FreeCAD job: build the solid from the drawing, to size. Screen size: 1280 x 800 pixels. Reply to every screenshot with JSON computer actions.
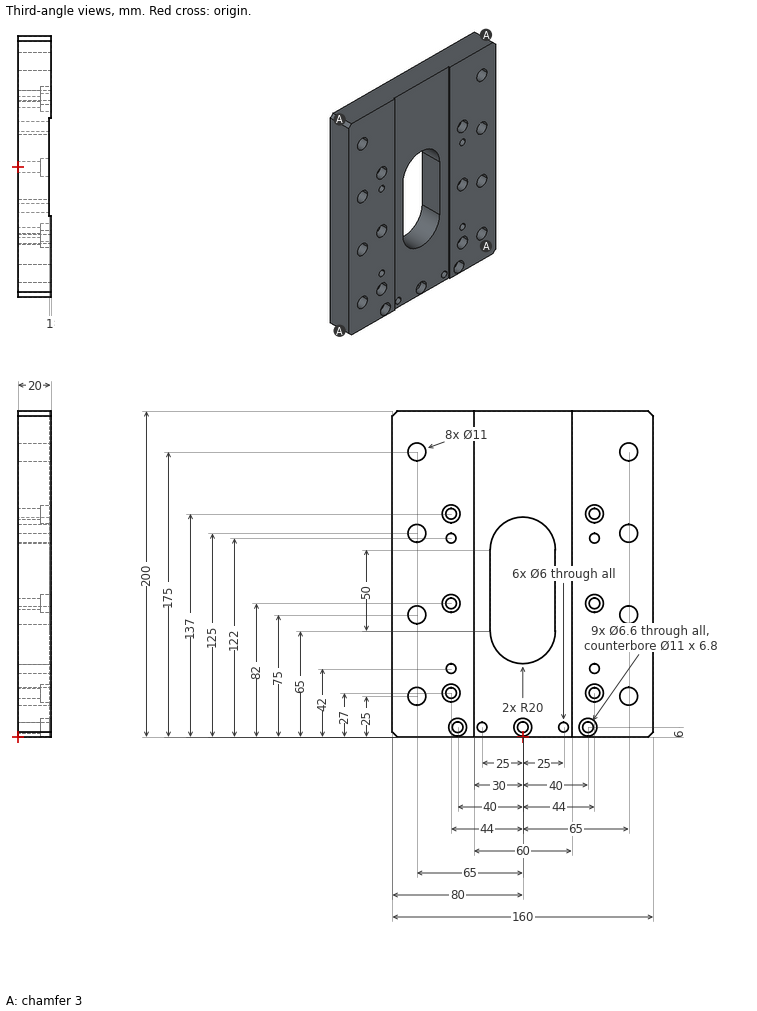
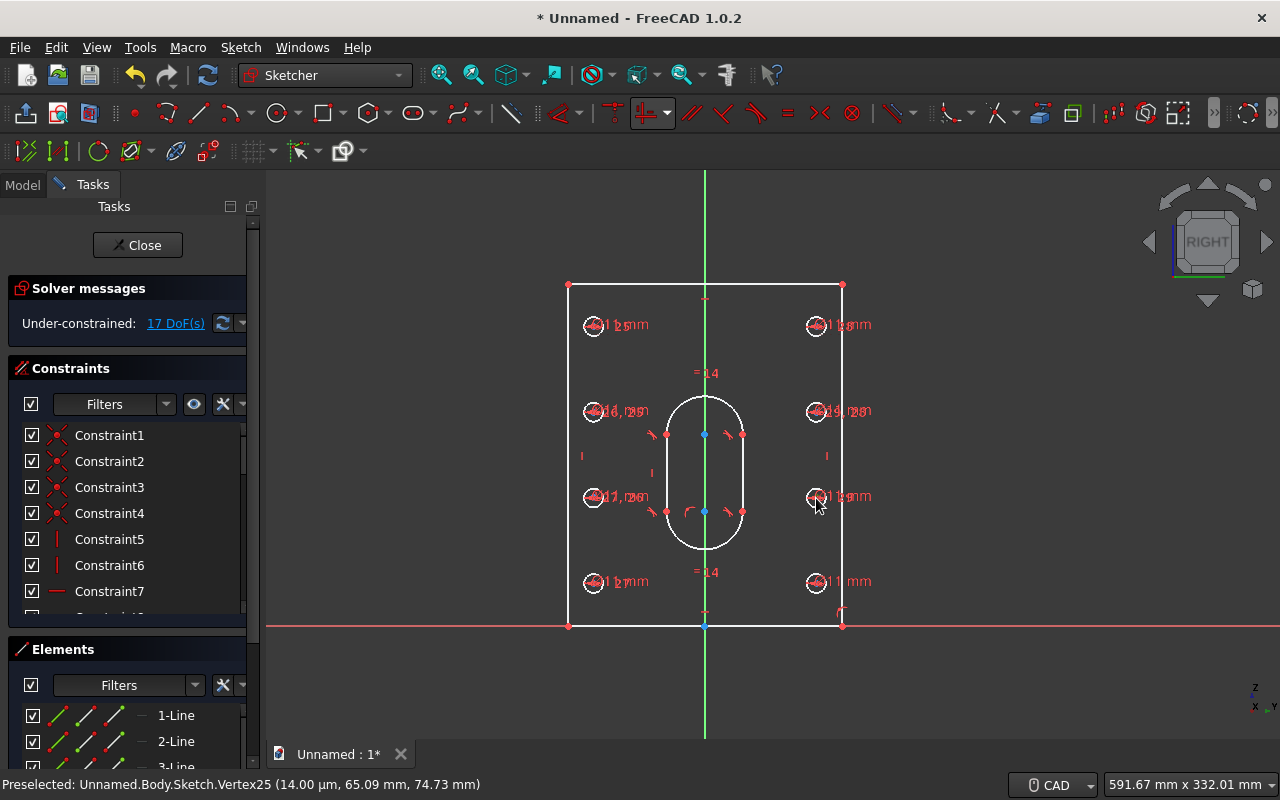
{"action": "left_click", "coordinate": [816, 583]}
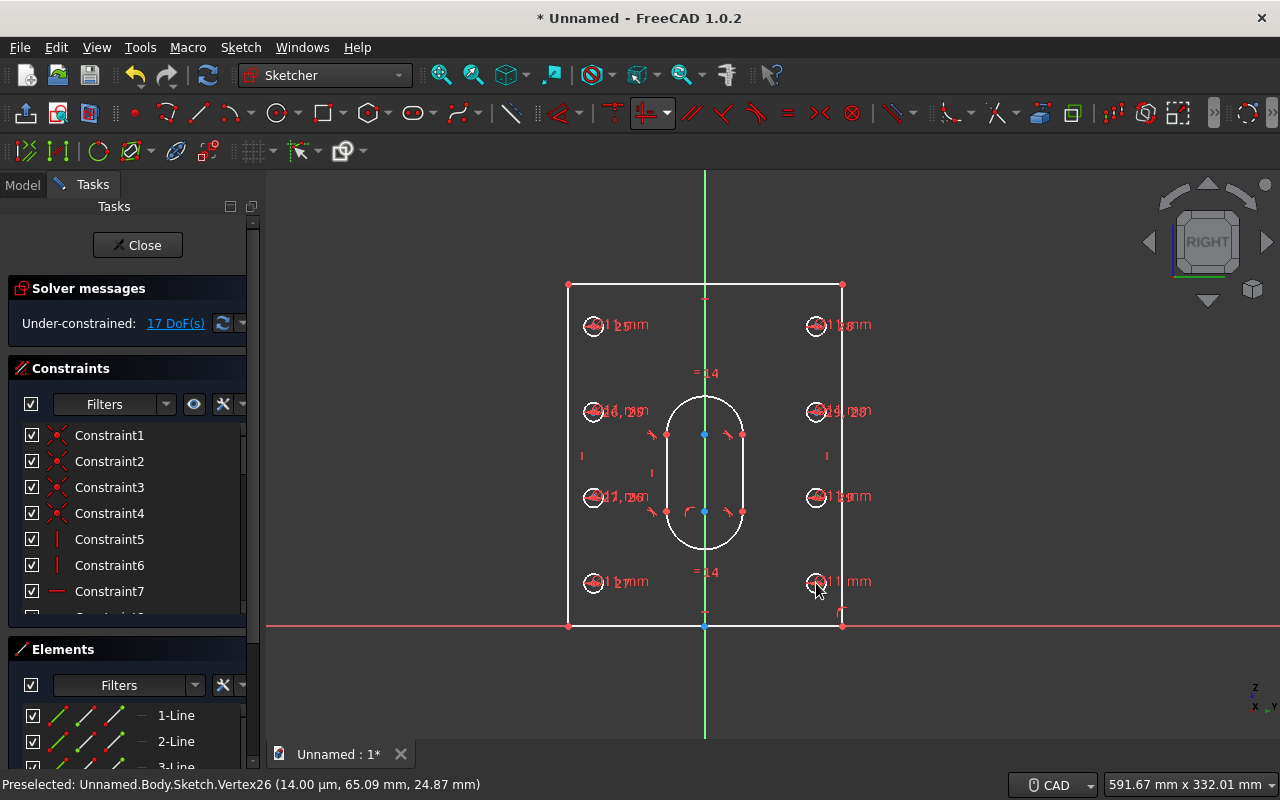
{"action": "key", "text": "v"}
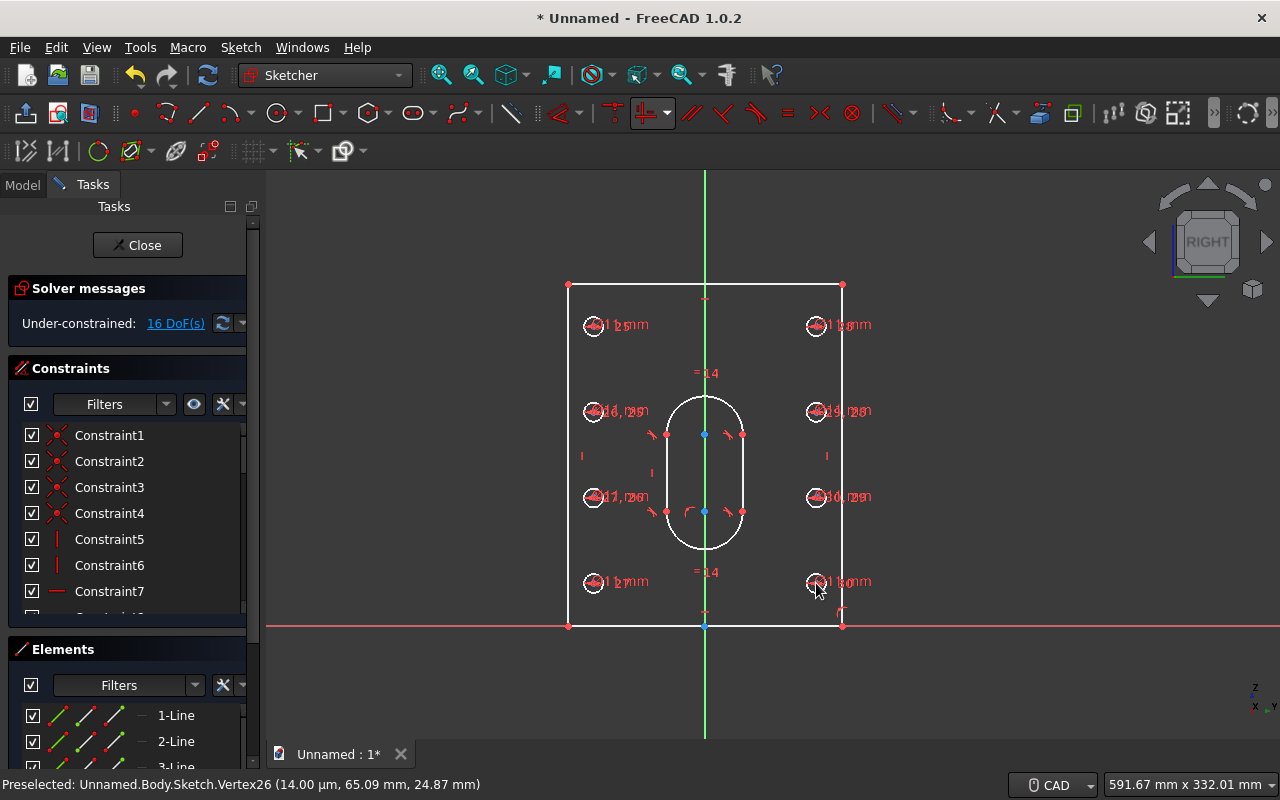
{"action": "key", "text": "d"}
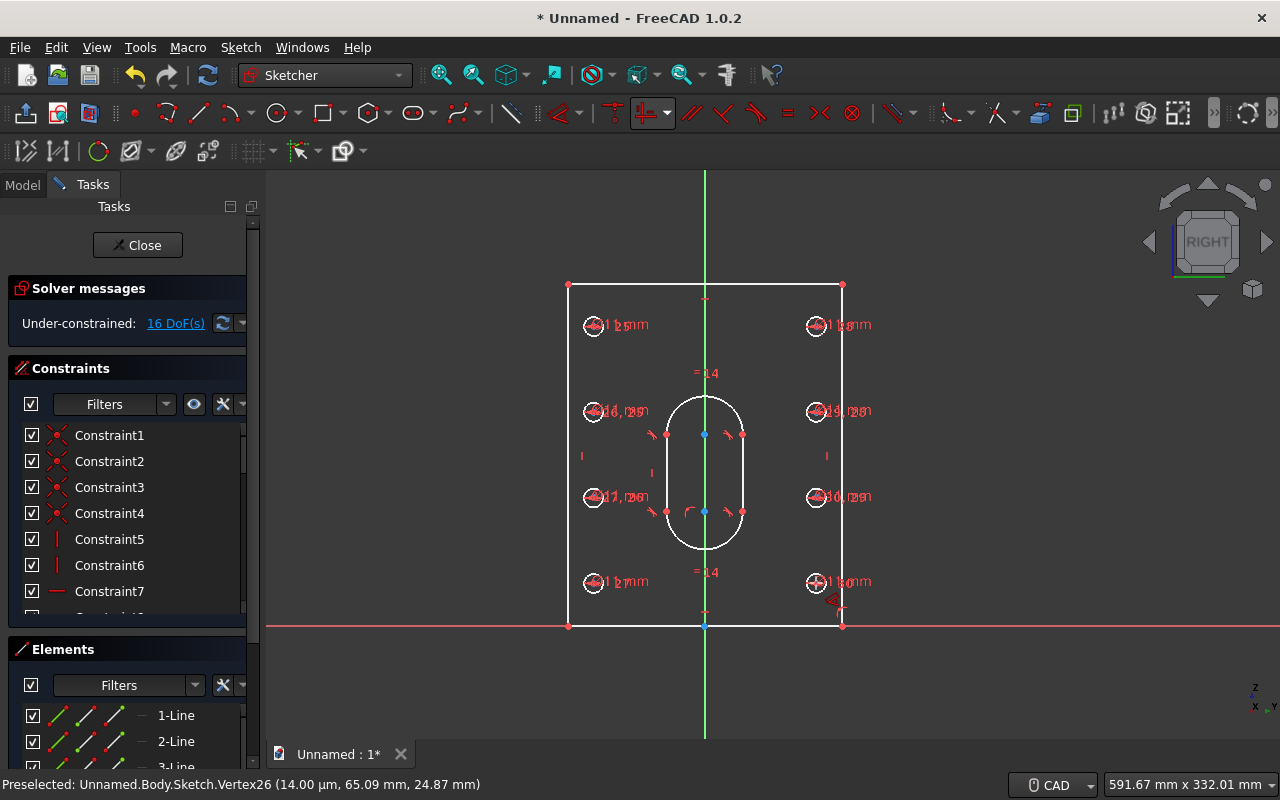
{"action": "left_click", "coordinate": [682, 542]}
{"action": "left_click", "coordinate": [663, 568]}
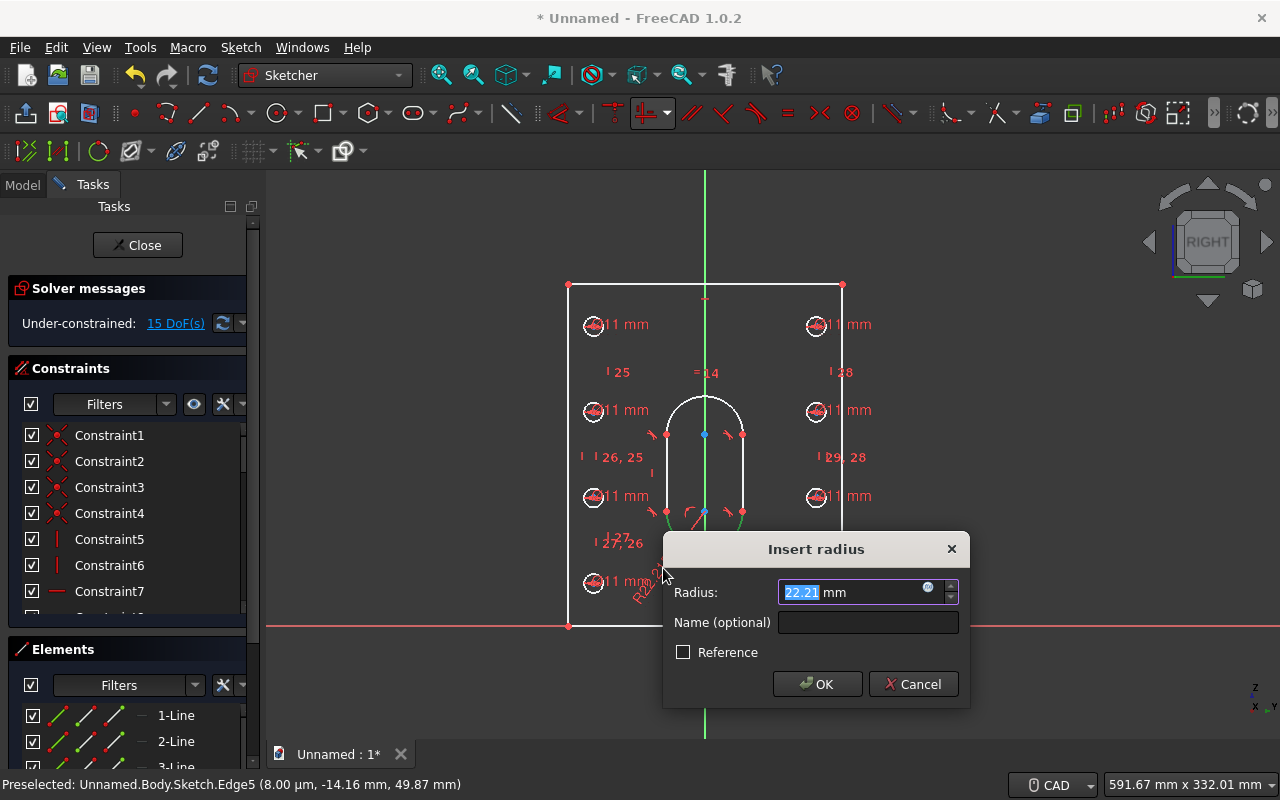
{"action": "type", "text": "20"}
{"action": "key", "text": "Return"}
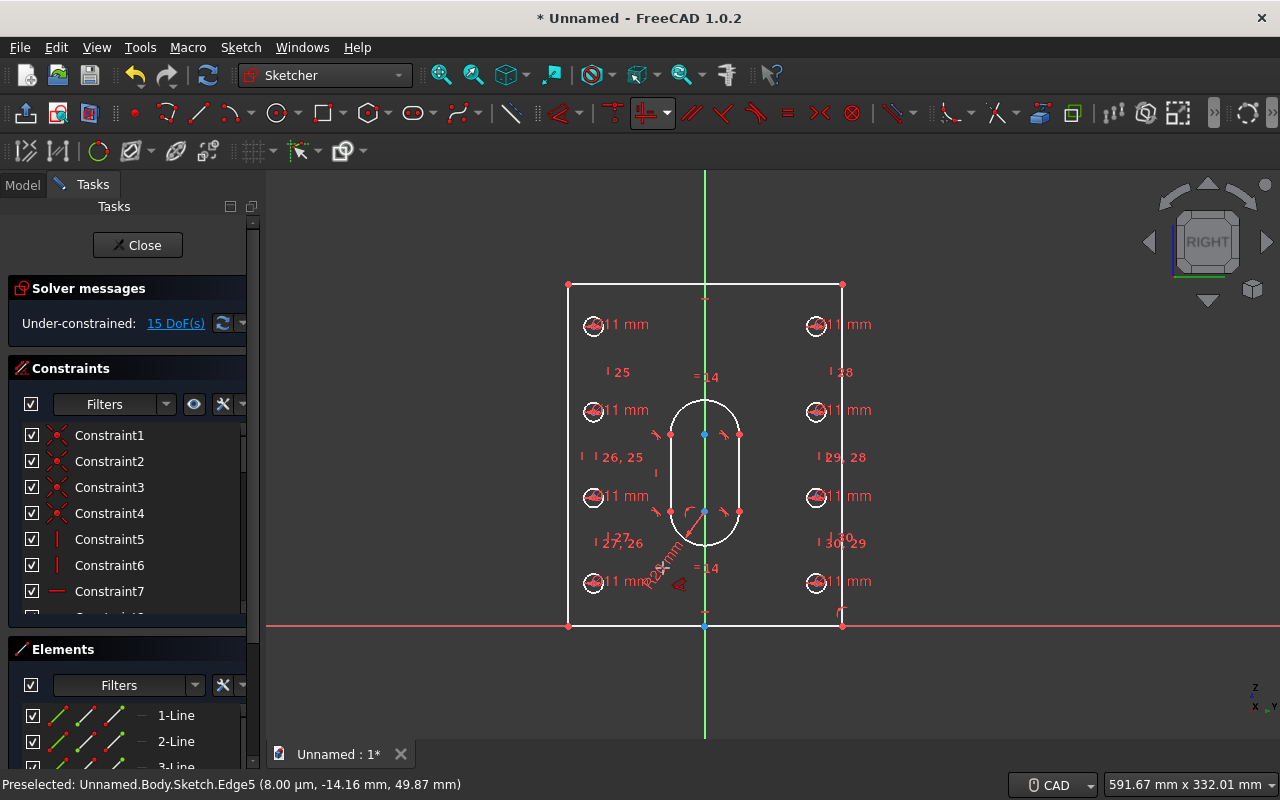
{"action": "left_click", "coordinate": [671, 488]}
{"action": "left_click", "coordinate": [637, 473]}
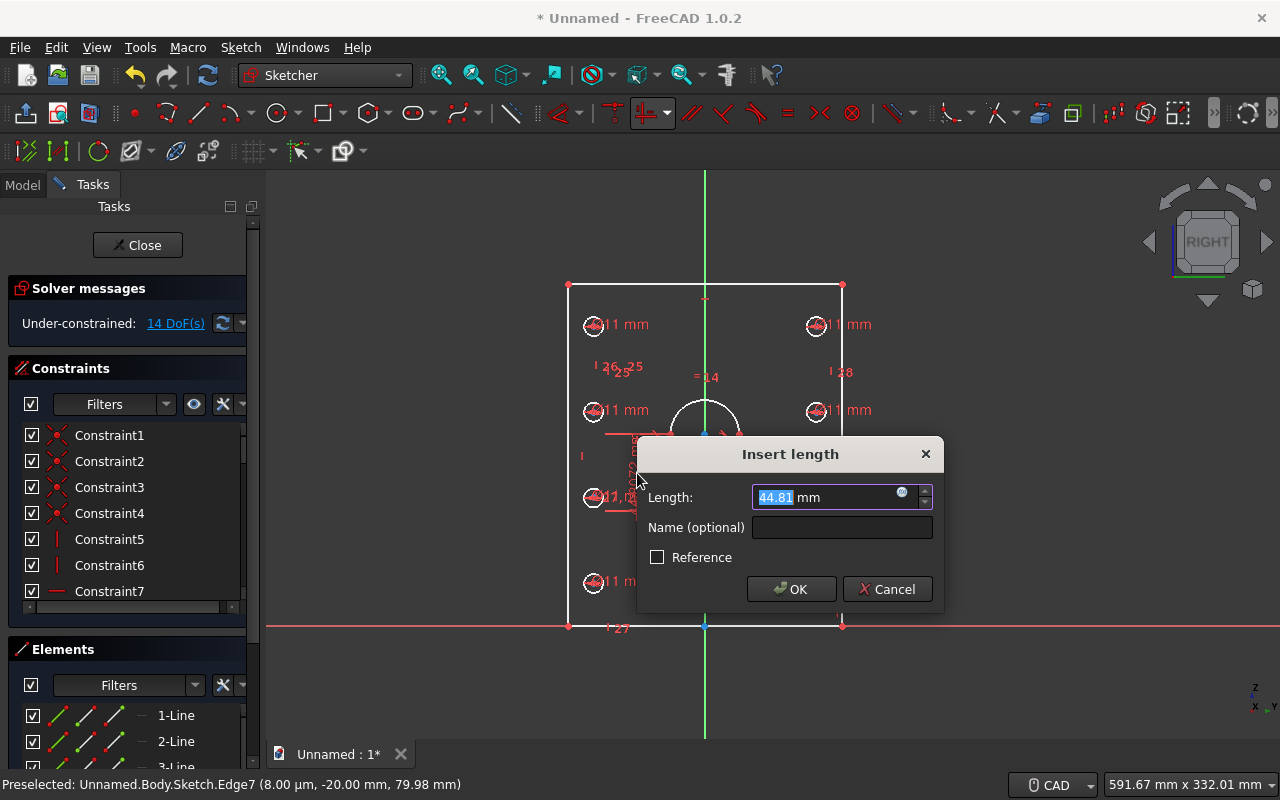
{"action": "type", "text": "50"}
{"action": "key", "text": "Return"}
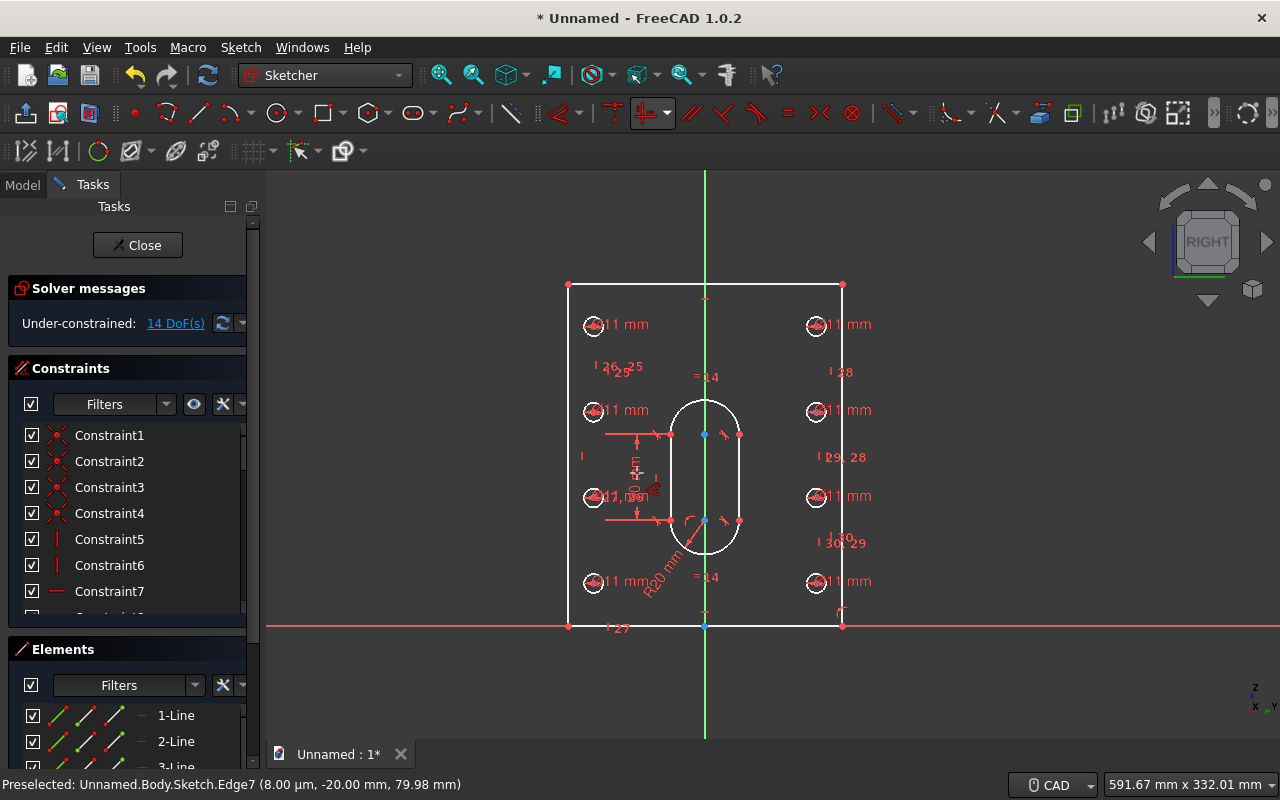
{"action": "left_click", "coordinate": [594, 327]}
{"action": "left_click", "coordinate": [649, 660]}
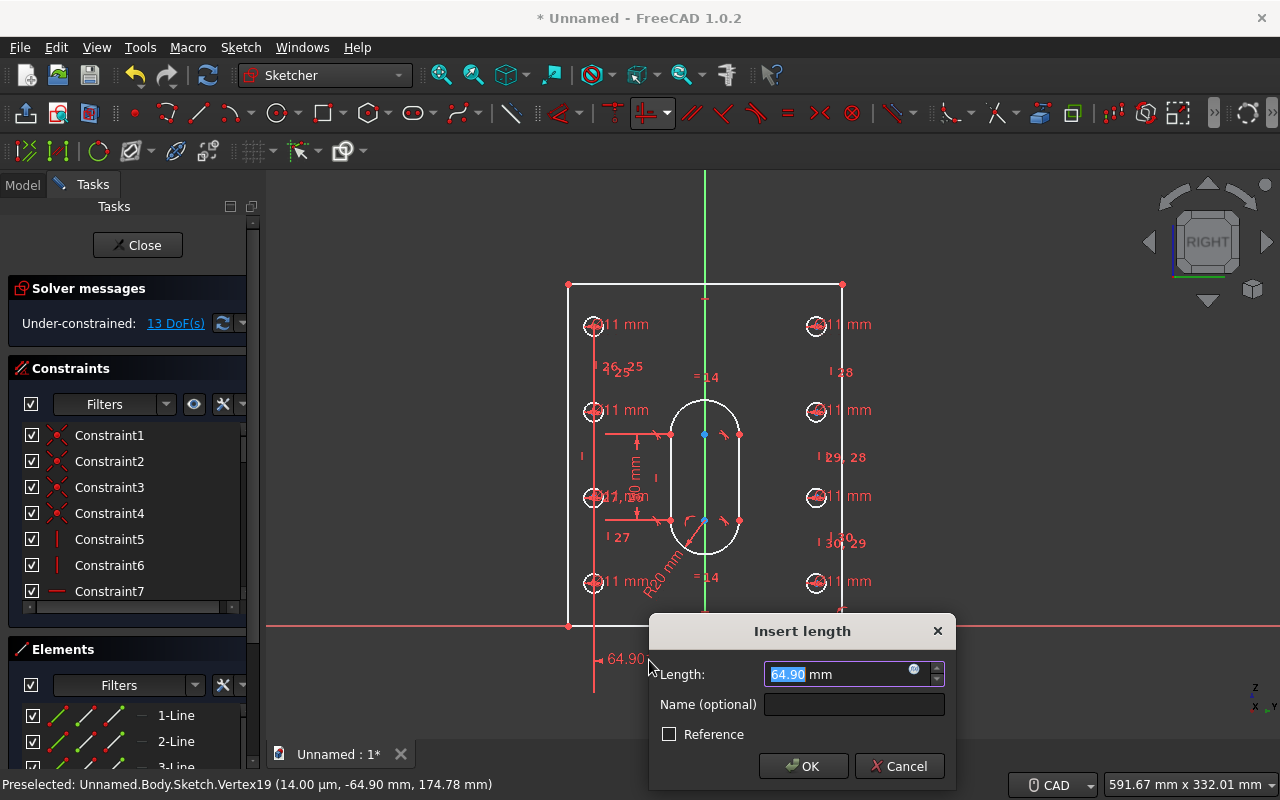
{"action": "type", "text": "65"}
{"action": "key", "text": "Return"}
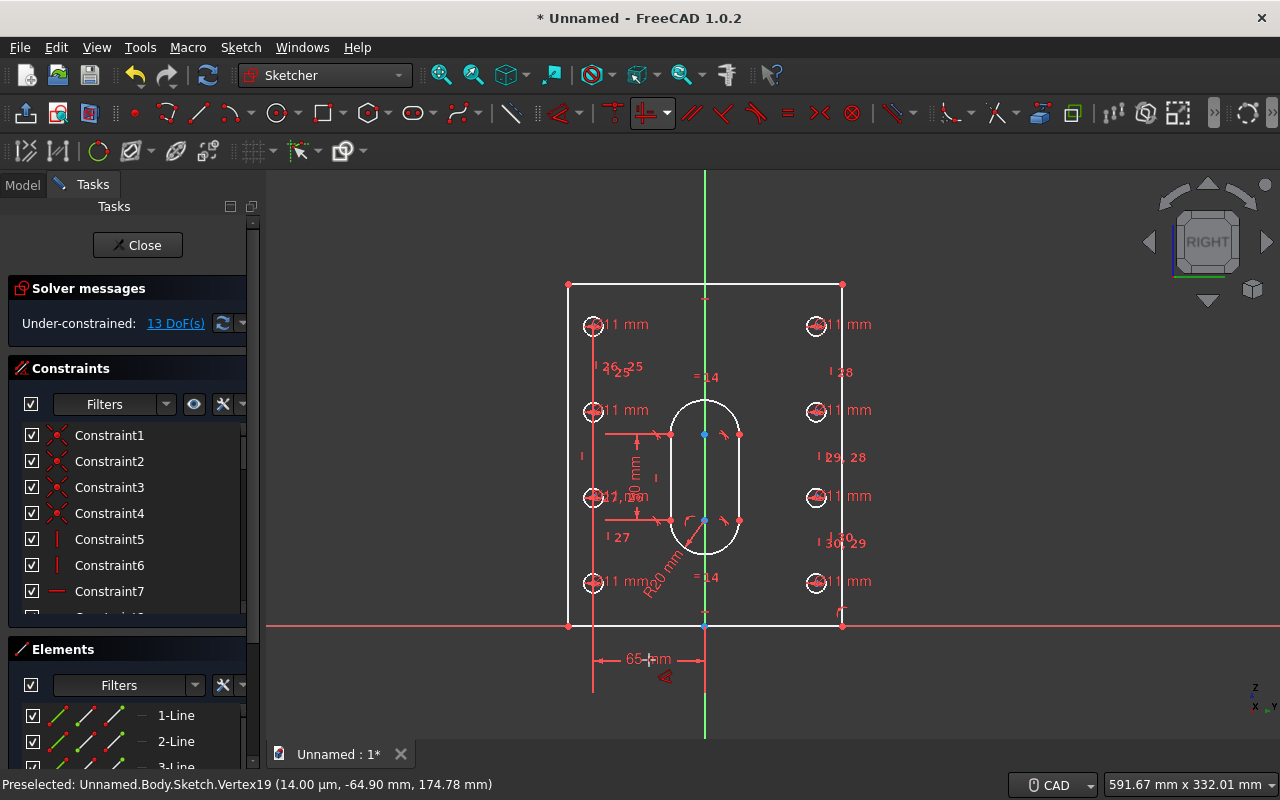
{"action": "left_click", "coordinate": [593, 498]}
{"action": "left_click", "coordinate": [739, 562]}